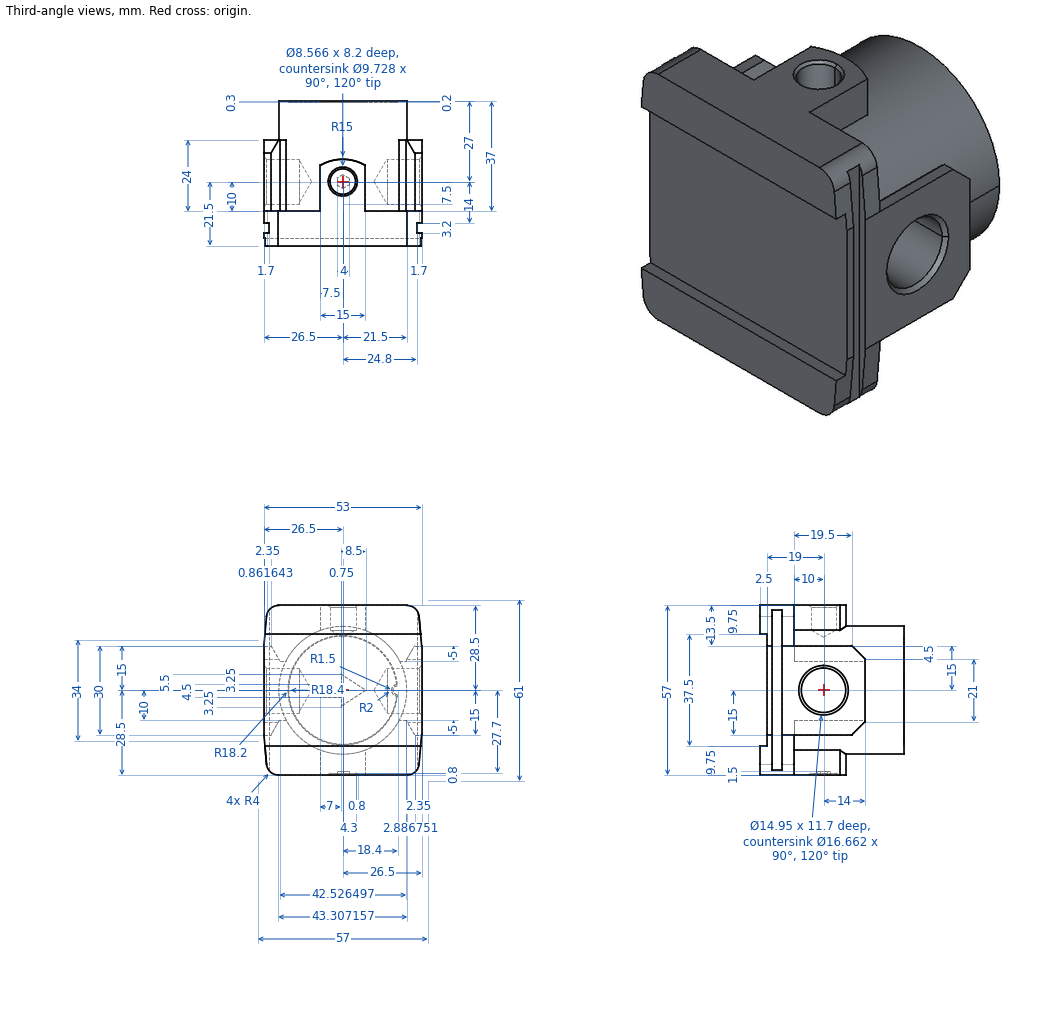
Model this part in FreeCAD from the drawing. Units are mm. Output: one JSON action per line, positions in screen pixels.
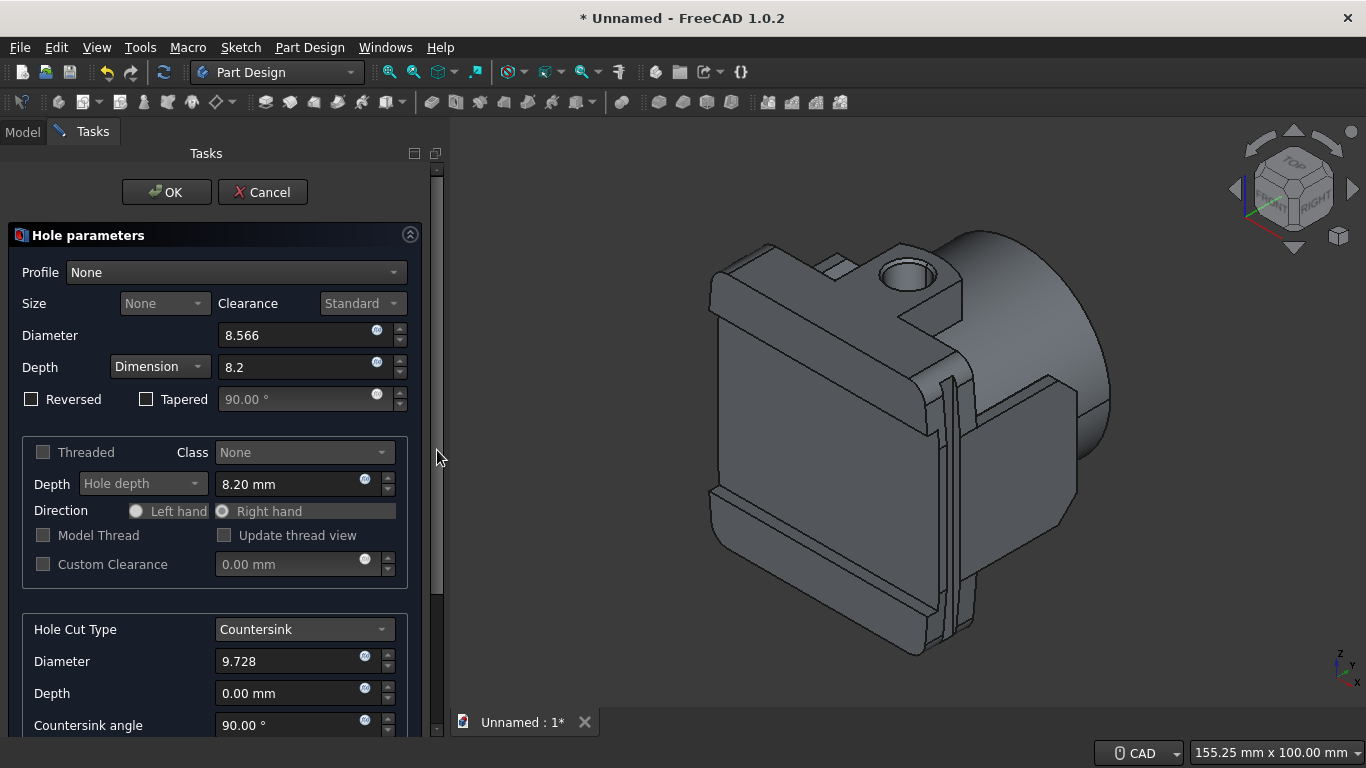
{"action": "left_click", "coordinate": [167, 192]}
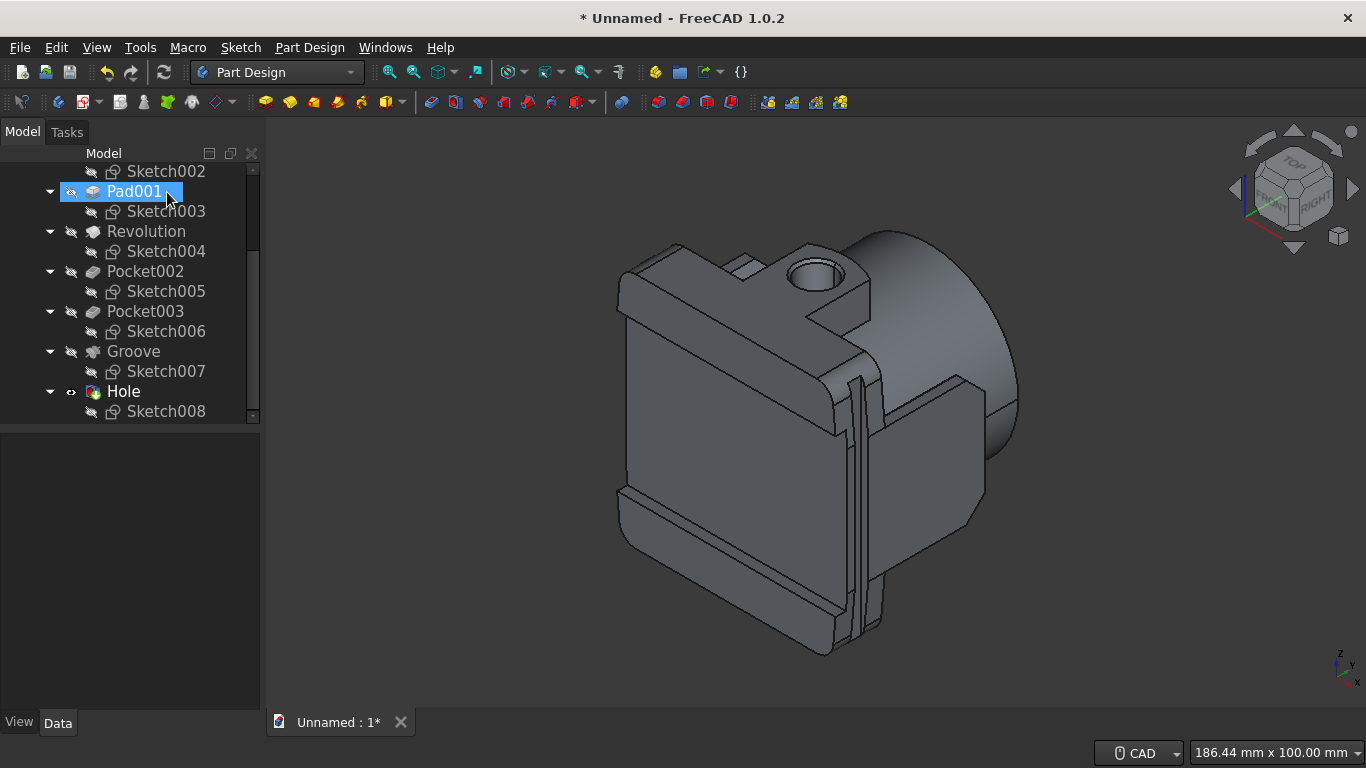
{"action": "key", "text": "5"}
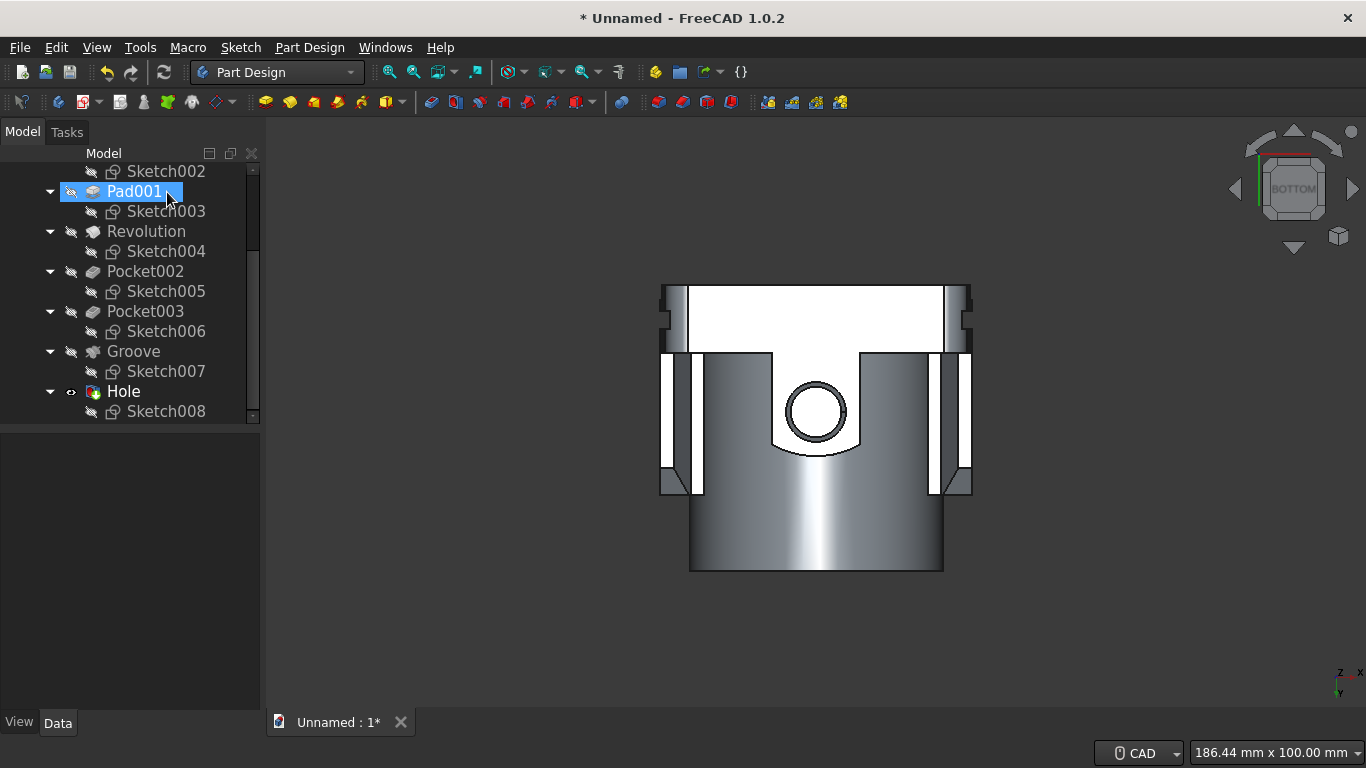
{"action": "left_click", "coordinate": [816, 321]}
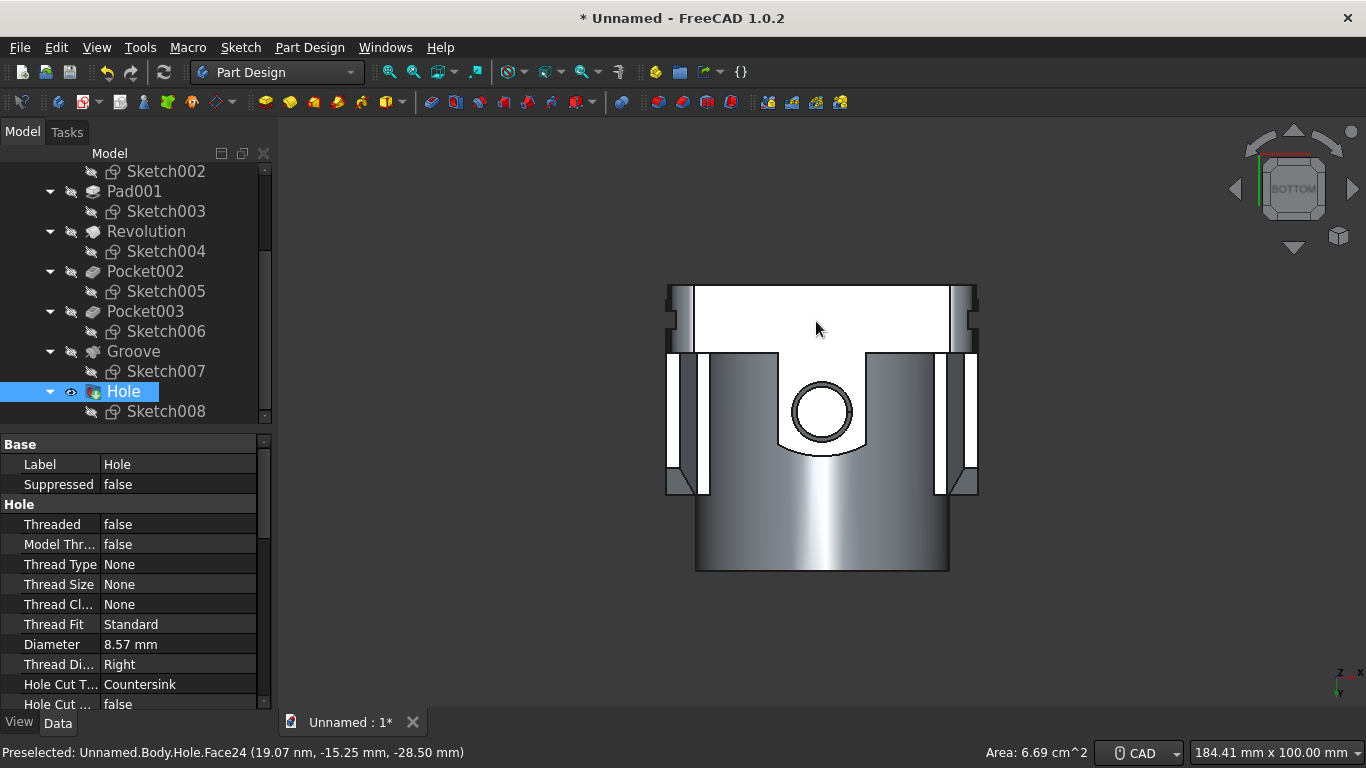
{"action": "left_click", "coordinate": [84, 102]}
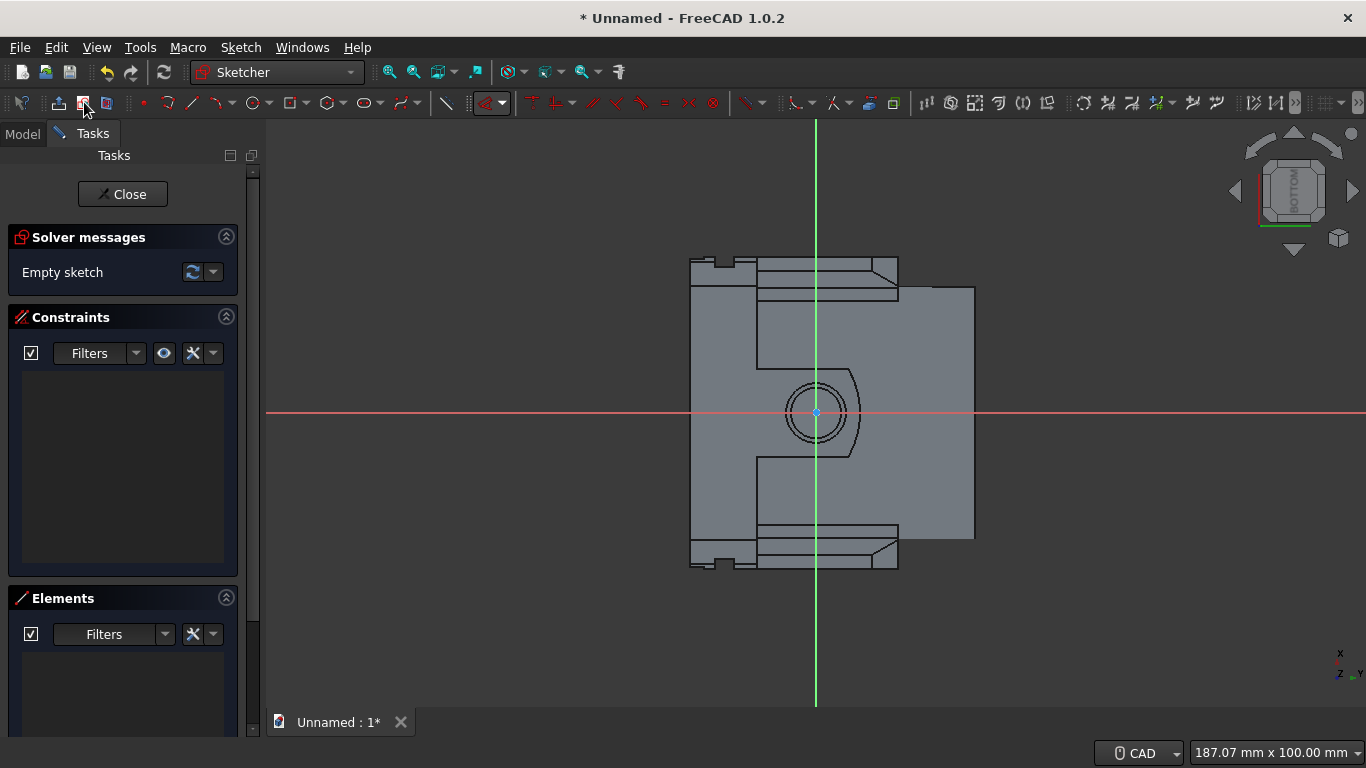
{"action": "scroll", "coordinate": [820, 413], "scroll_direction": "up", "scroll_amount": 14}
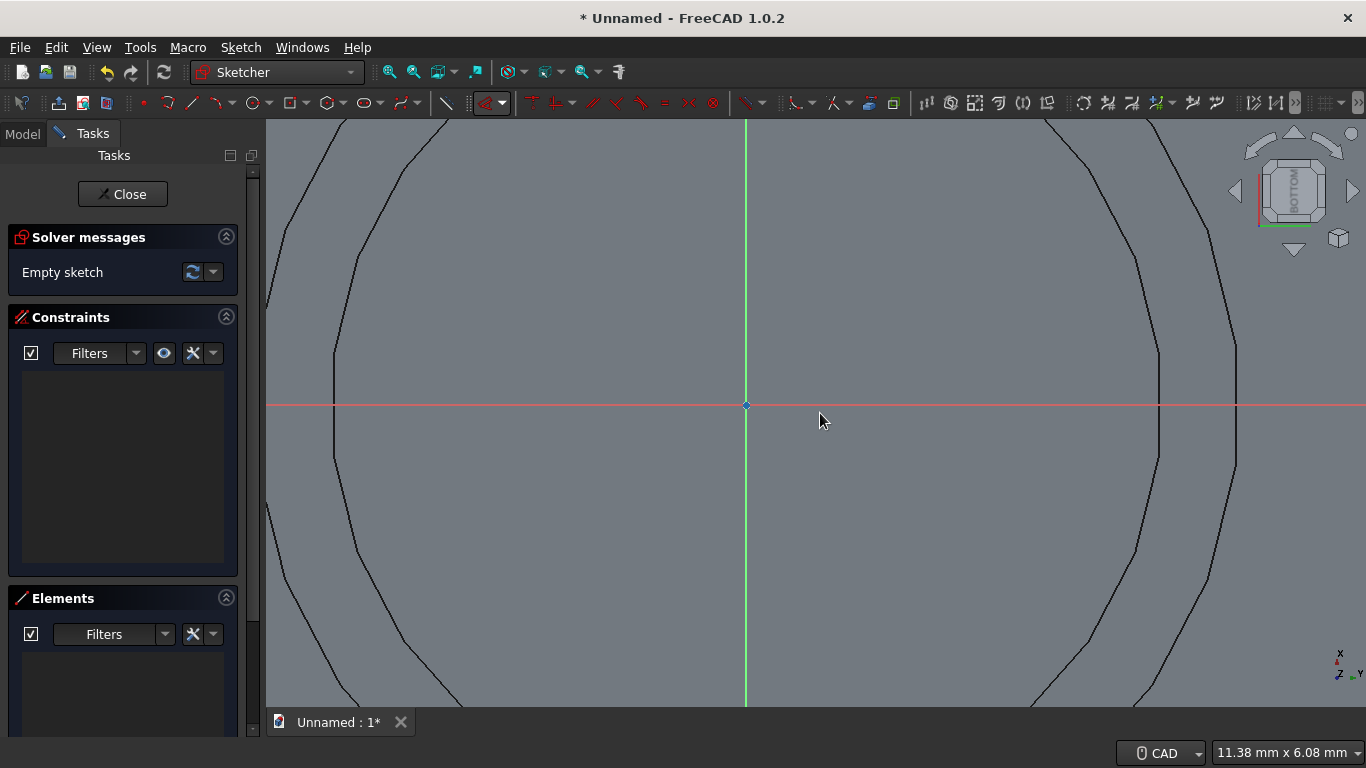
{"action": "left_click", "coordinate": [328, 104]}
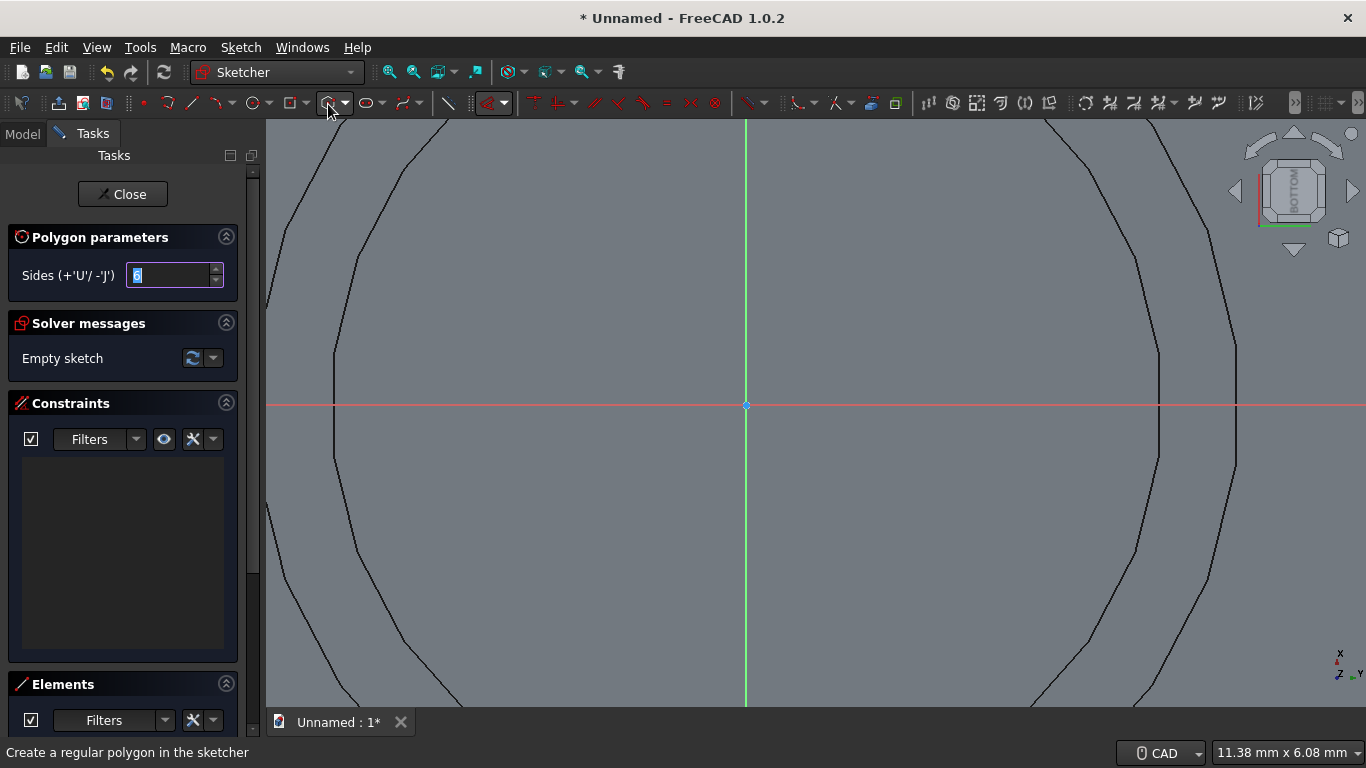
{"action": "left_click", "coordinate": [746, 405]}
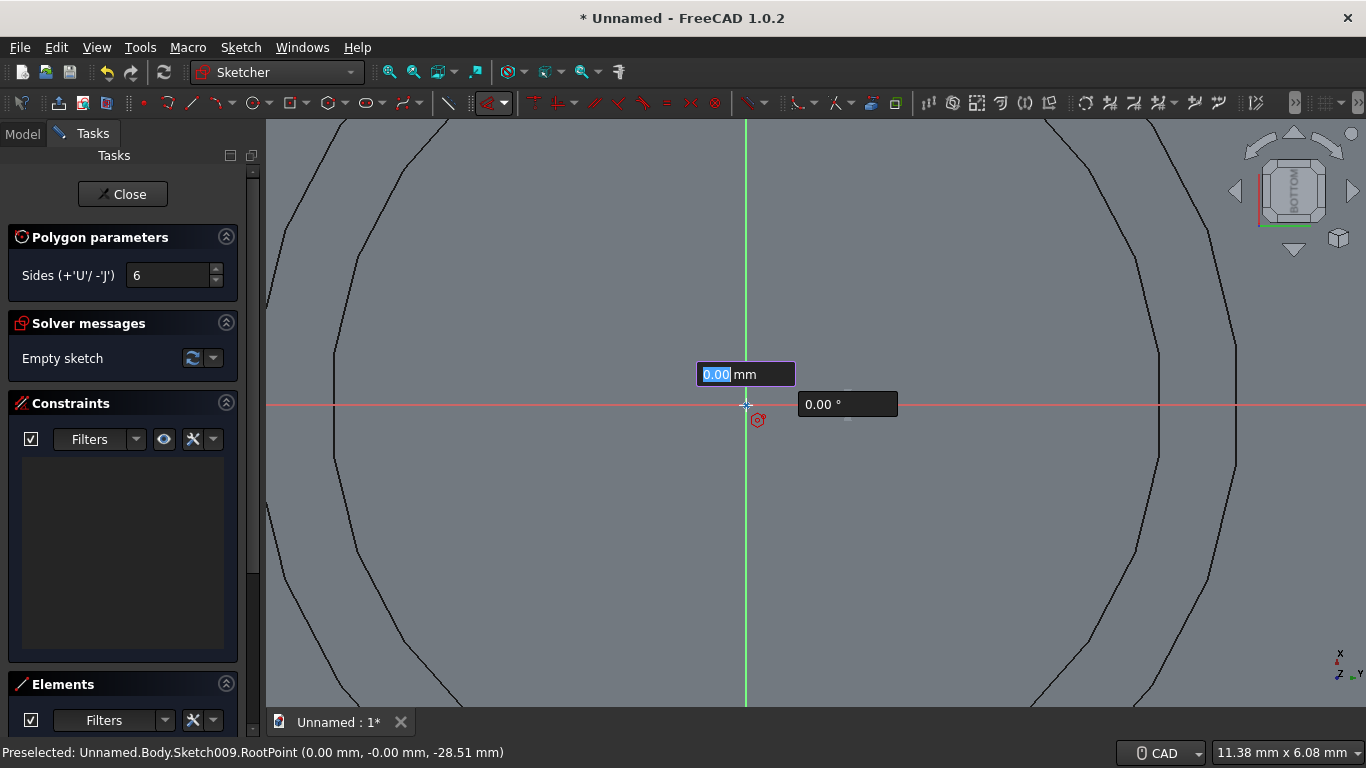
{"action": "left_click", "coordinate": [523, 405]}
{"action": "right_click", "coordinate": [523, 405]}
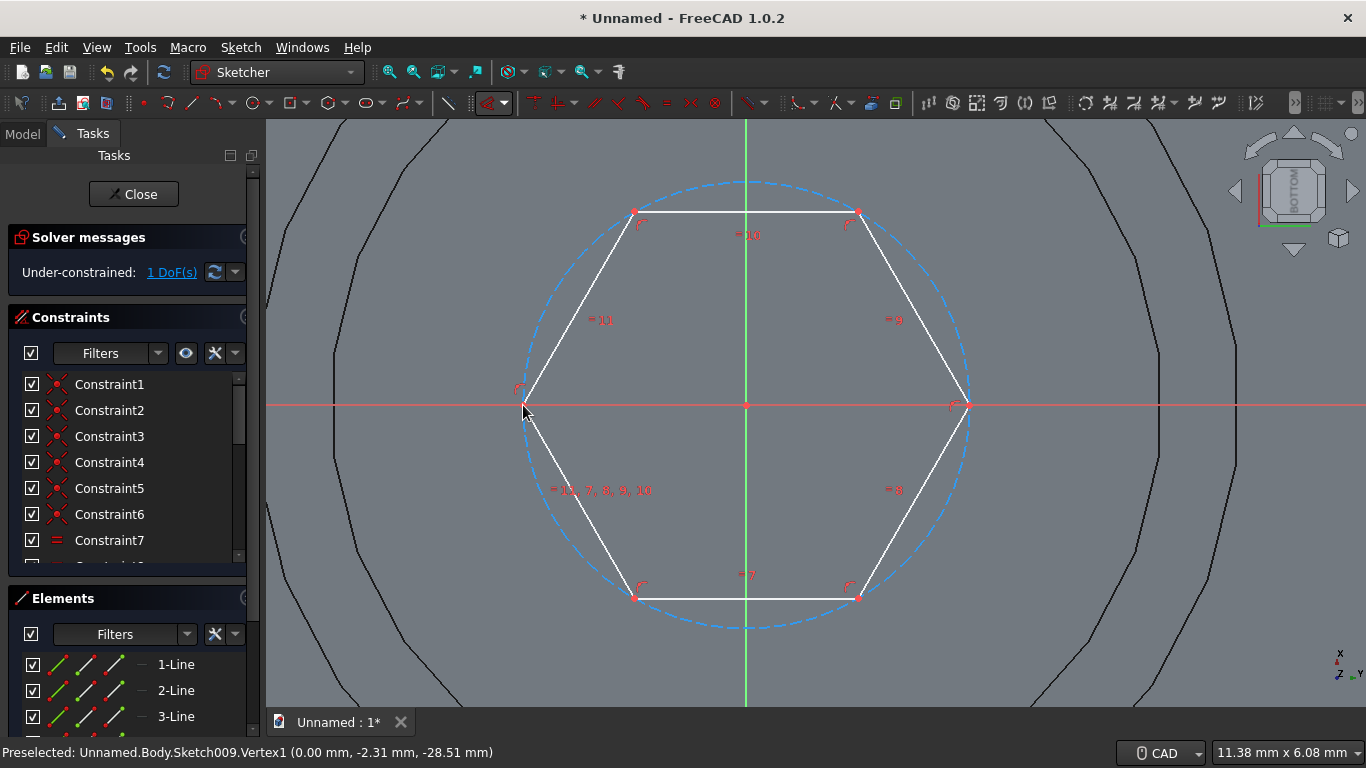
{"action": "left_click", "coordinate": [635, 599]}